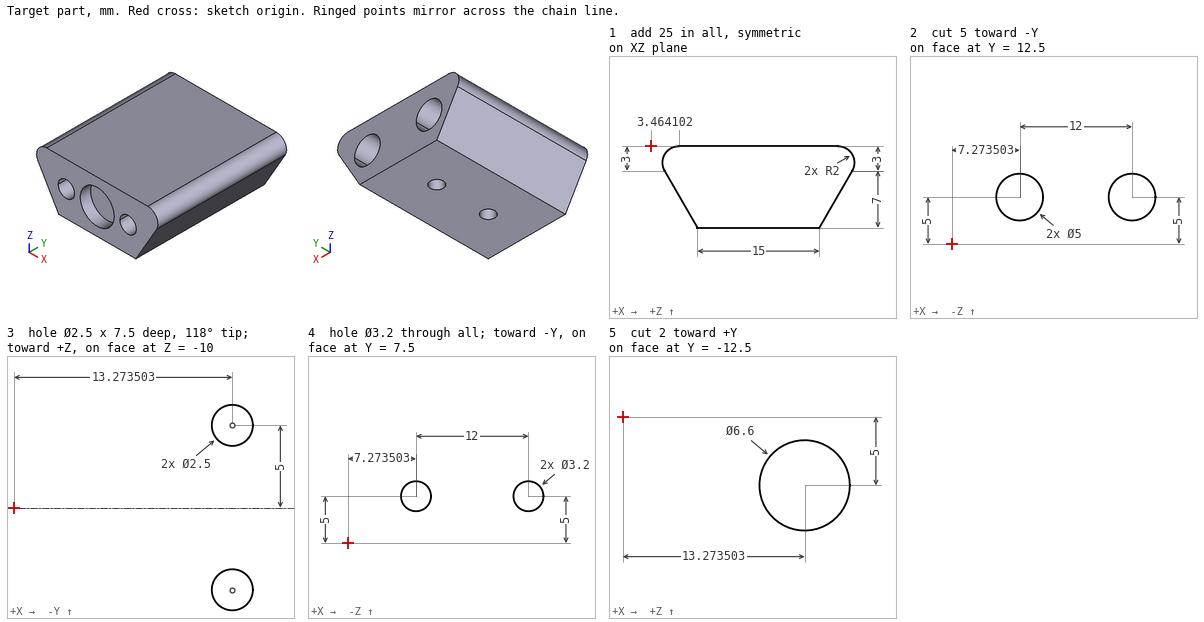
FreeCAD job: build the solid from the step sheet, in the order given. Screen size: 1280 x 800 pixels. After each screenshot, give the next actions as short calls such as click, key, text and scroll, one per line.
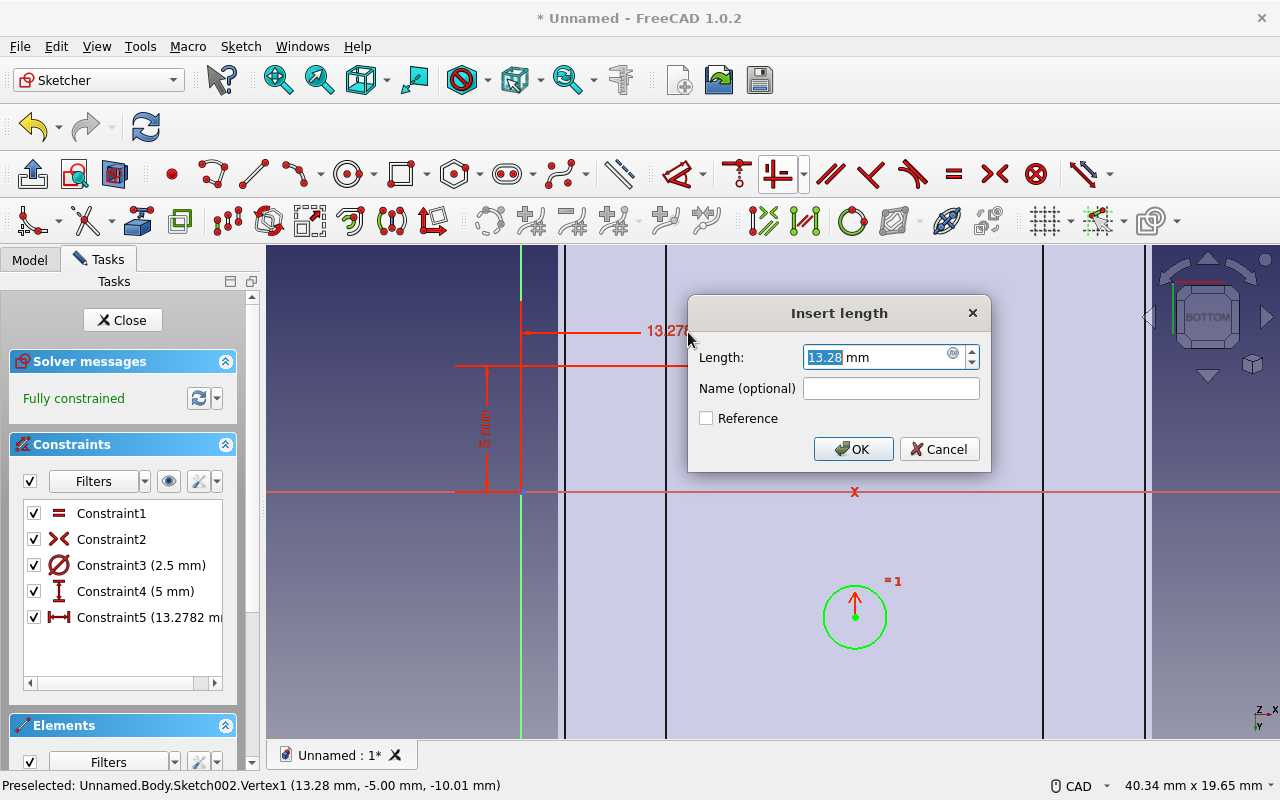
text(13.273503)
key(Return)
key(Escape)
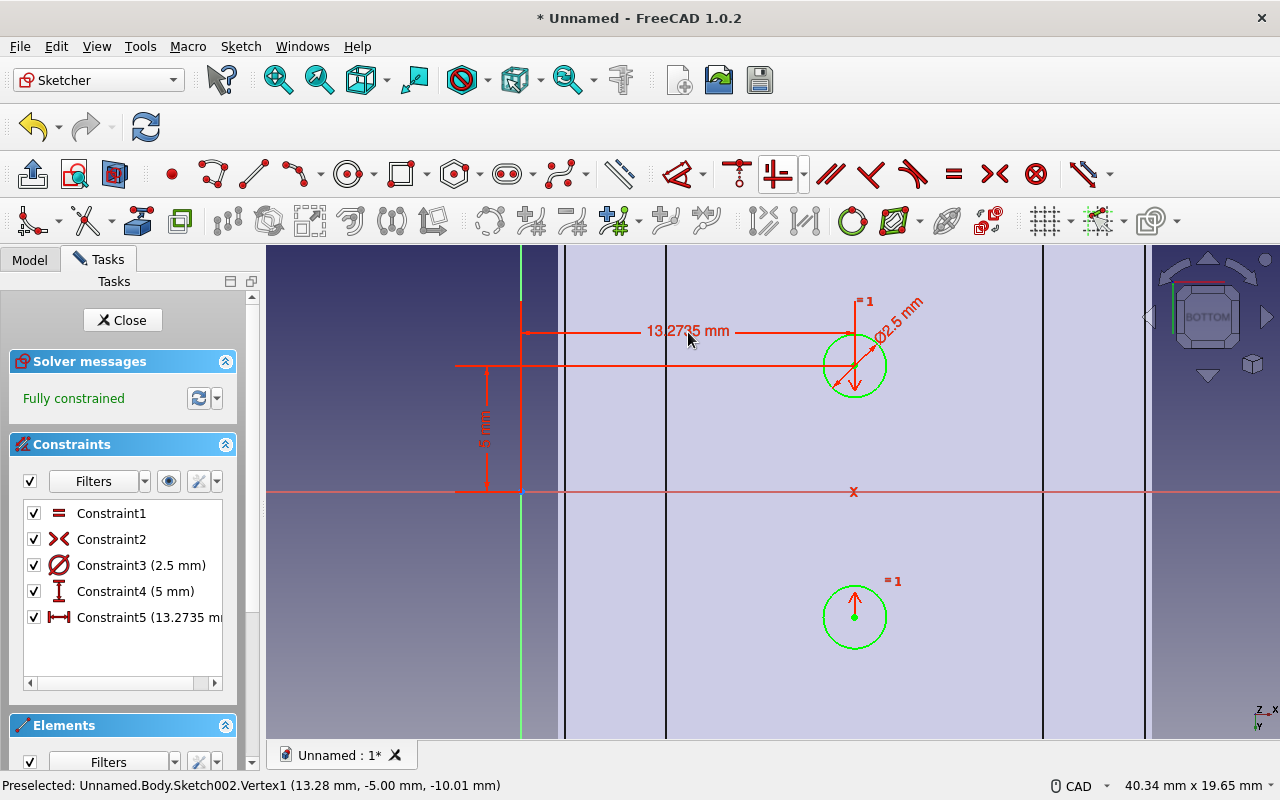
click(123, 320)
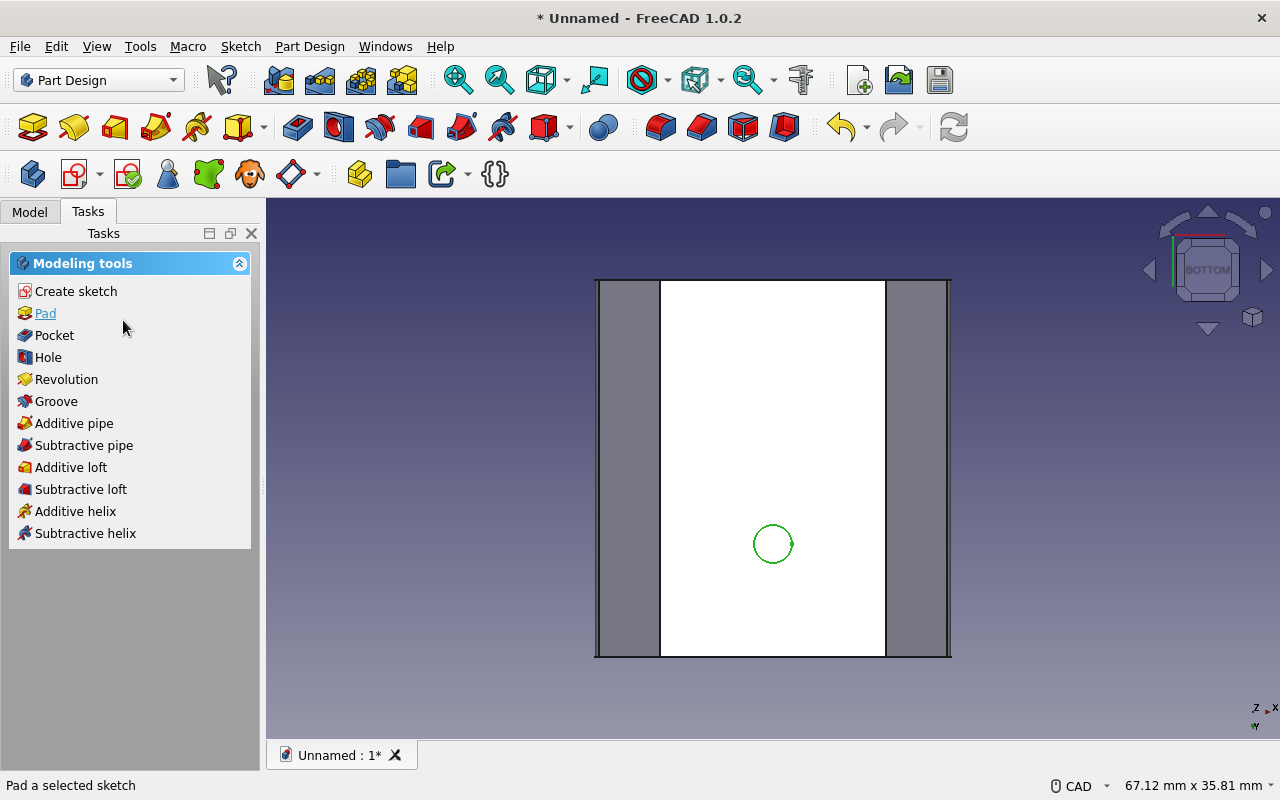
click(339, 128)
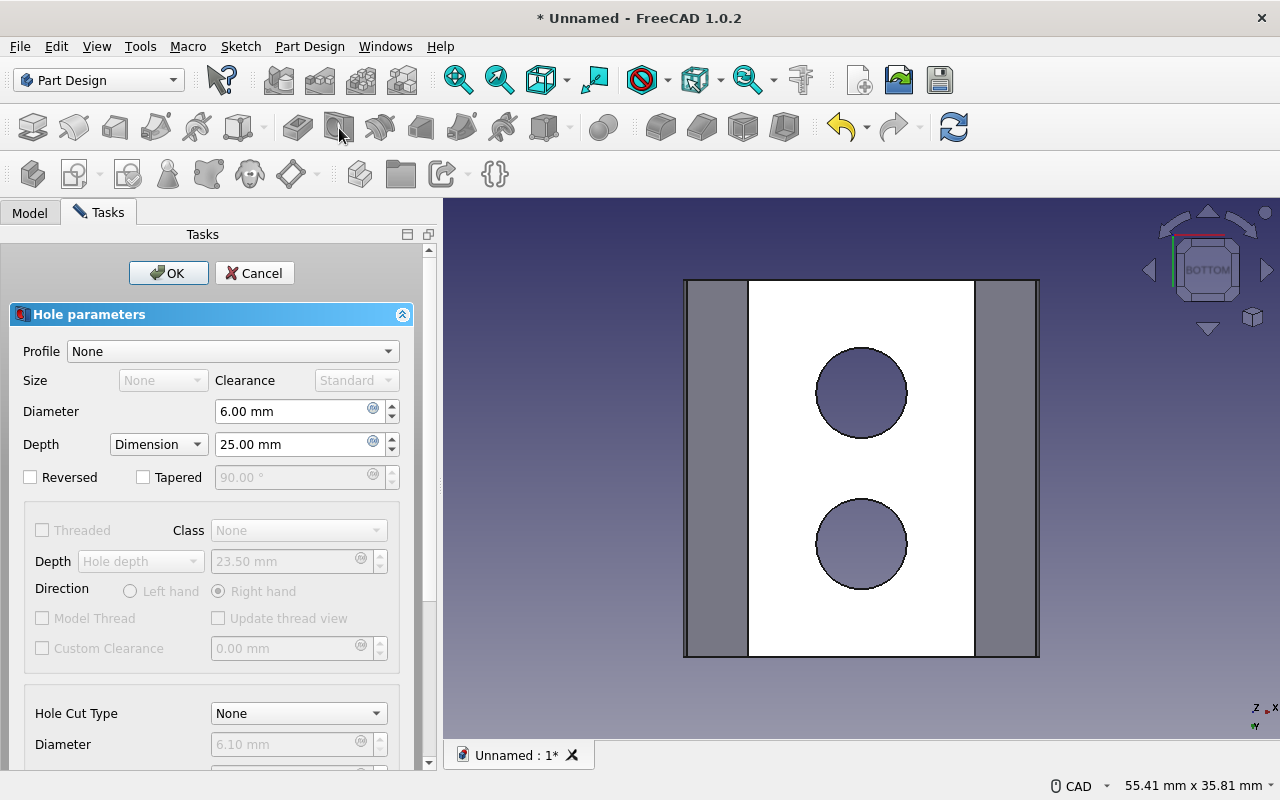
triple_click(300, 412)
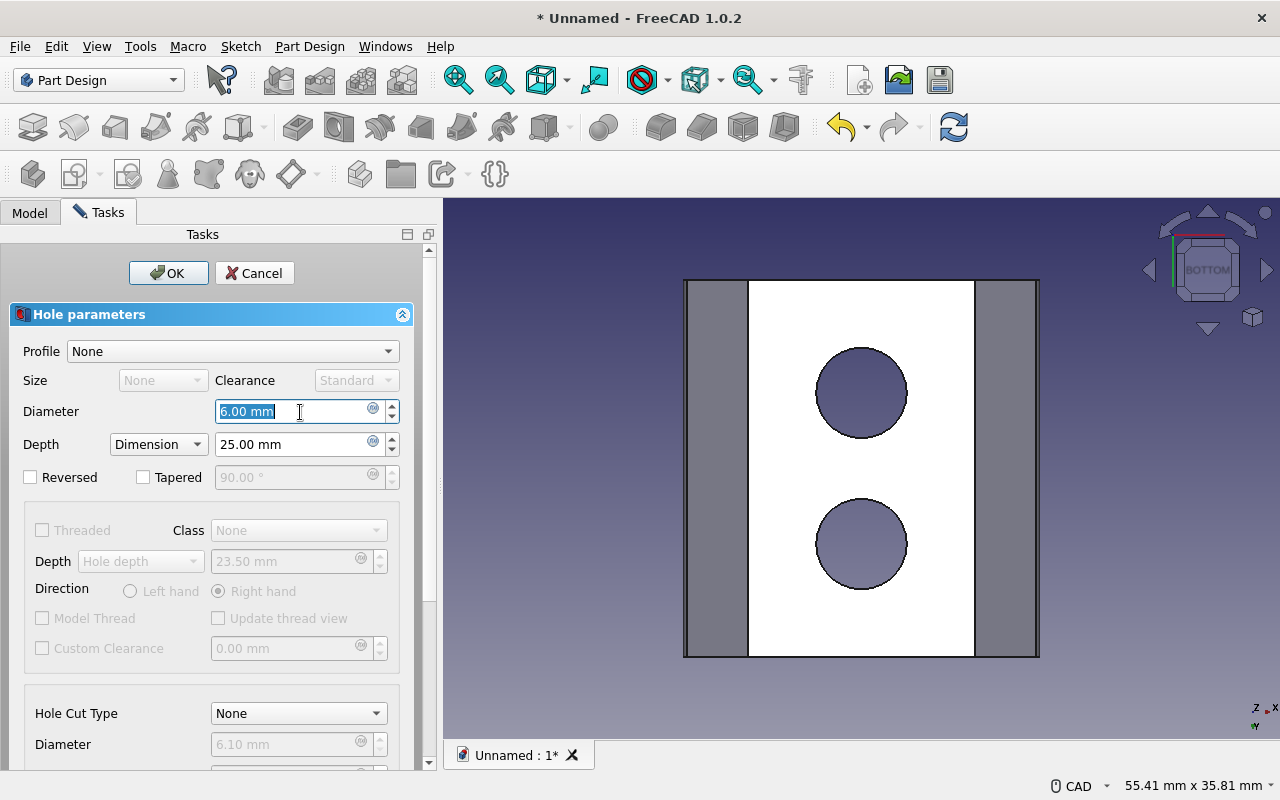
text(2.5)
key(Tab)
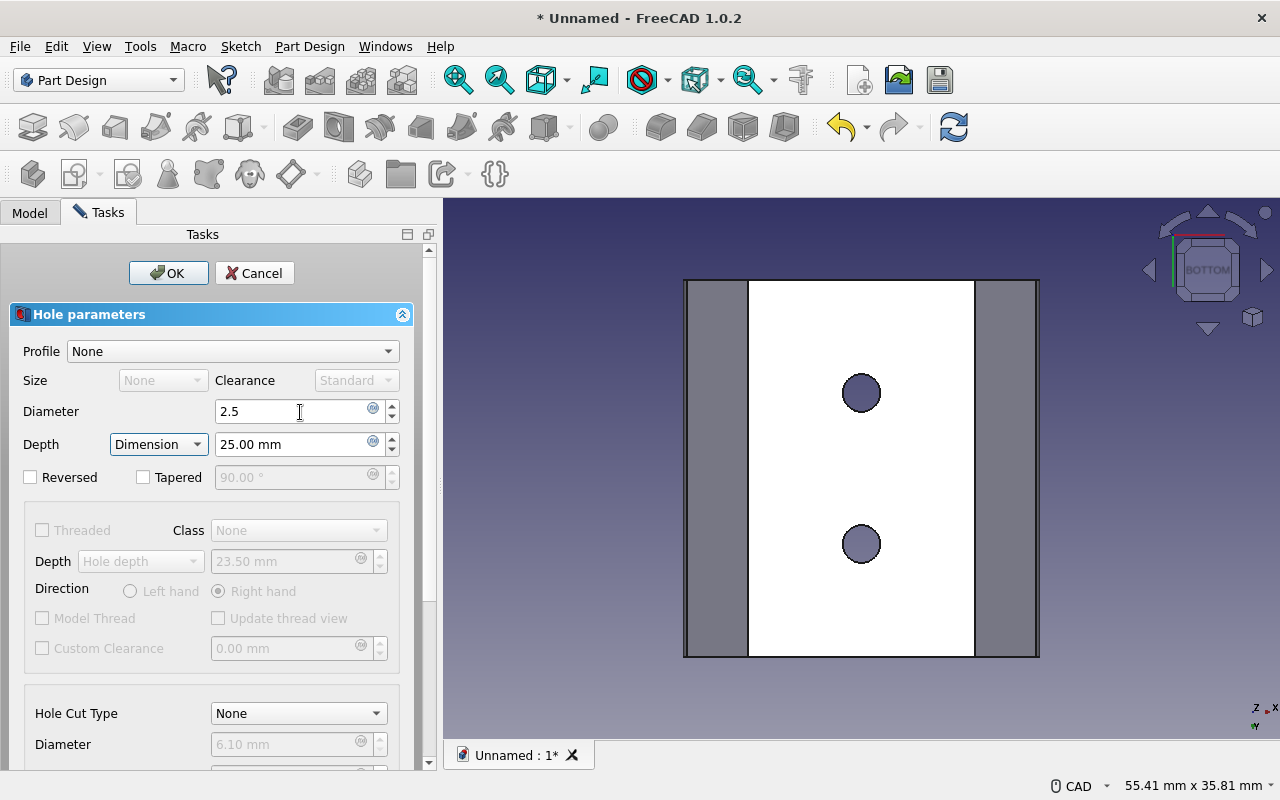
triple_click(300, 444)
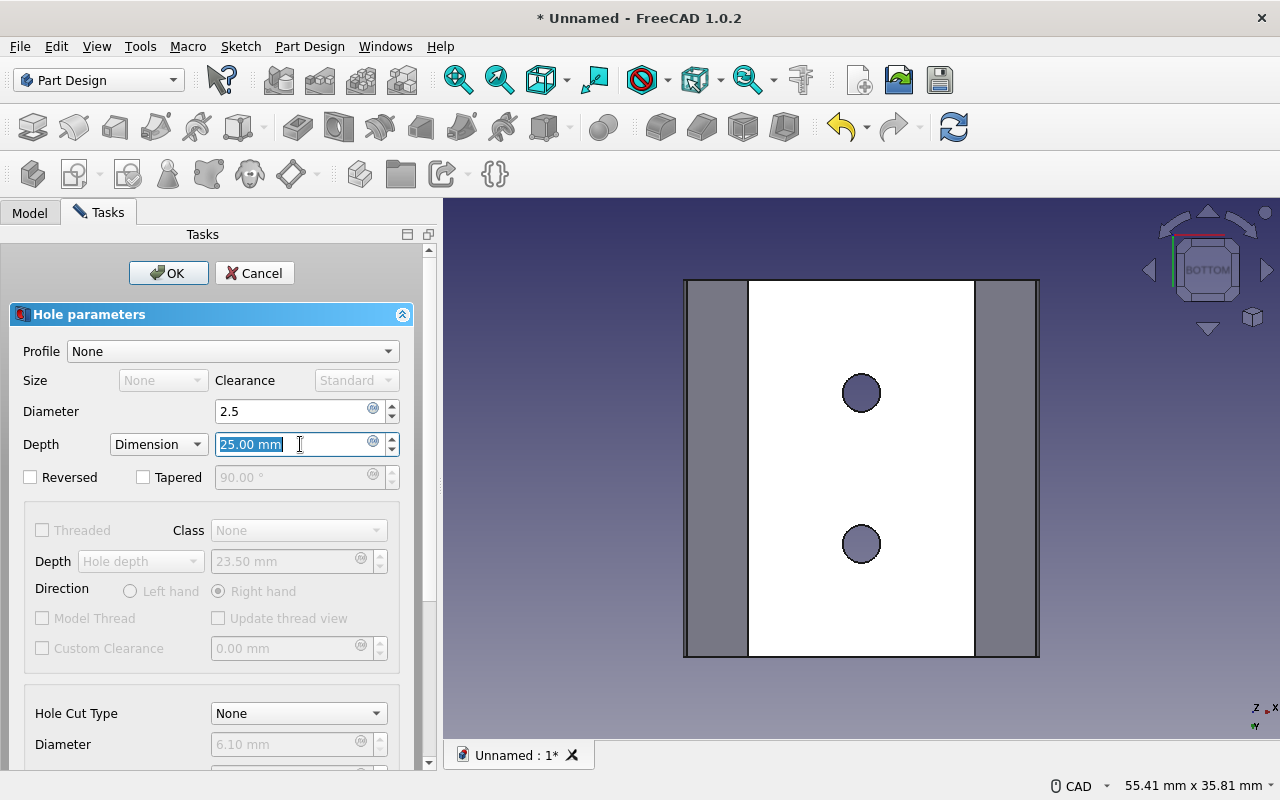
text(7.5)
key(Tab)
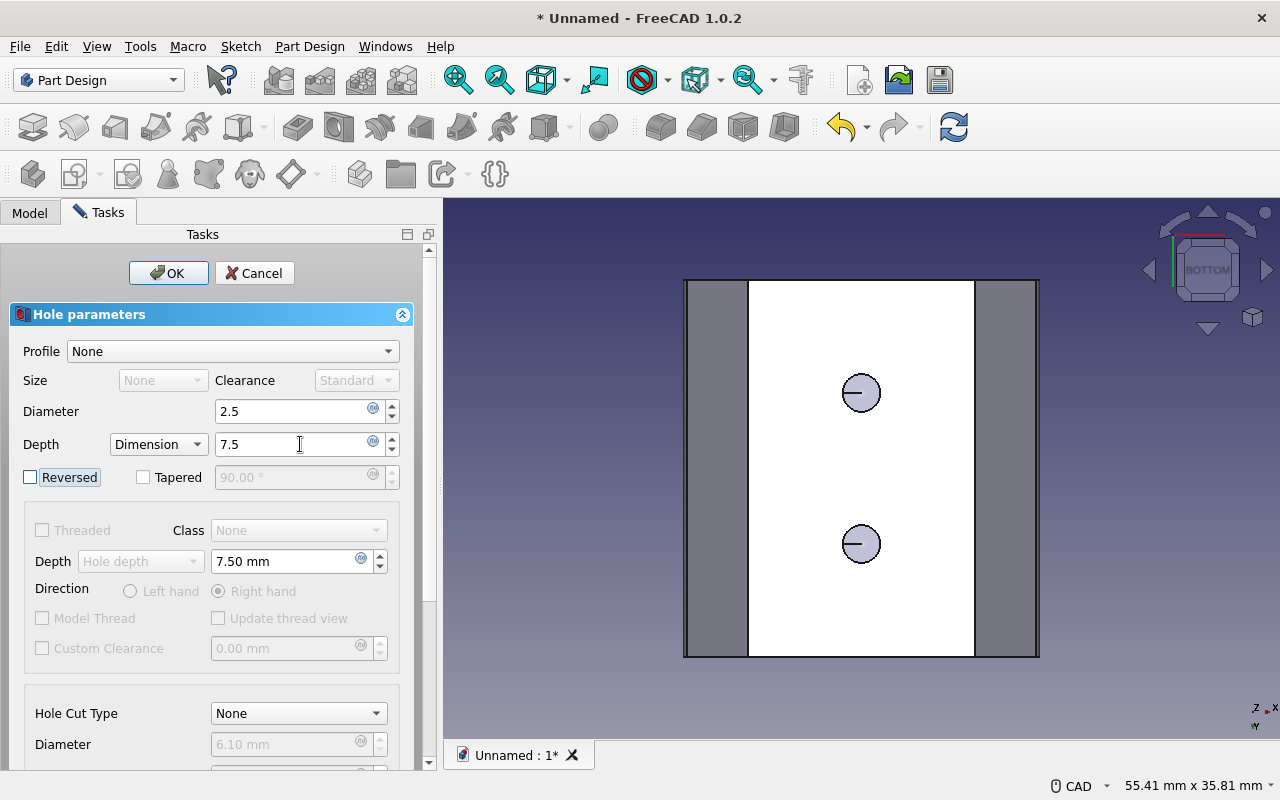
click(169, 273)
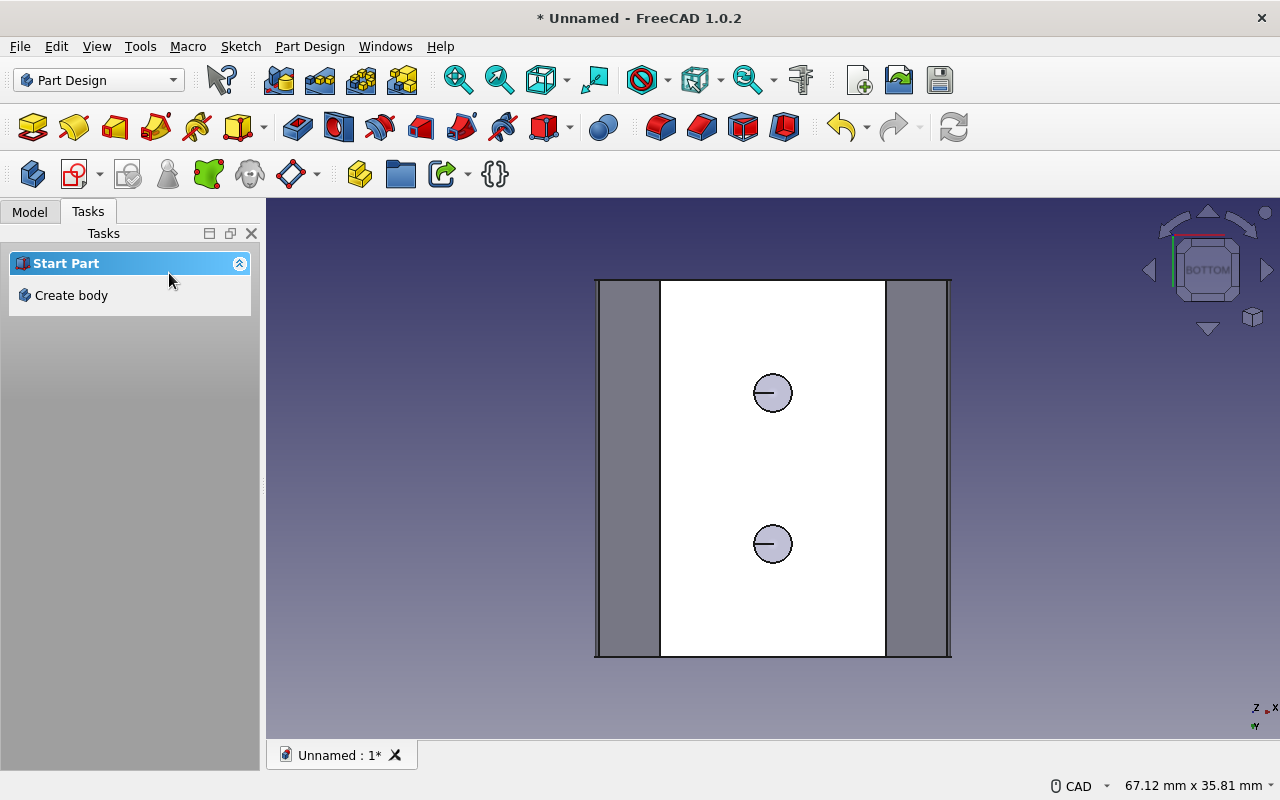
key(4)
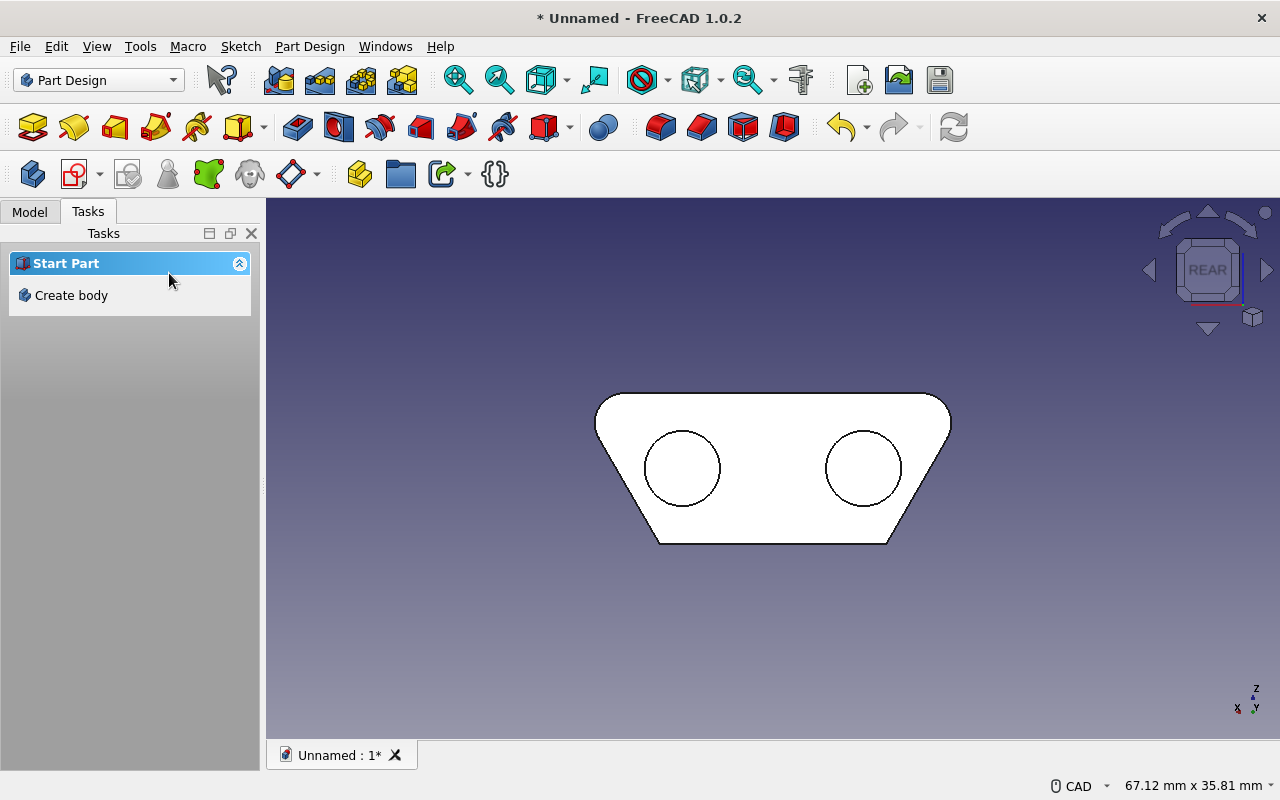
click(459, 80)